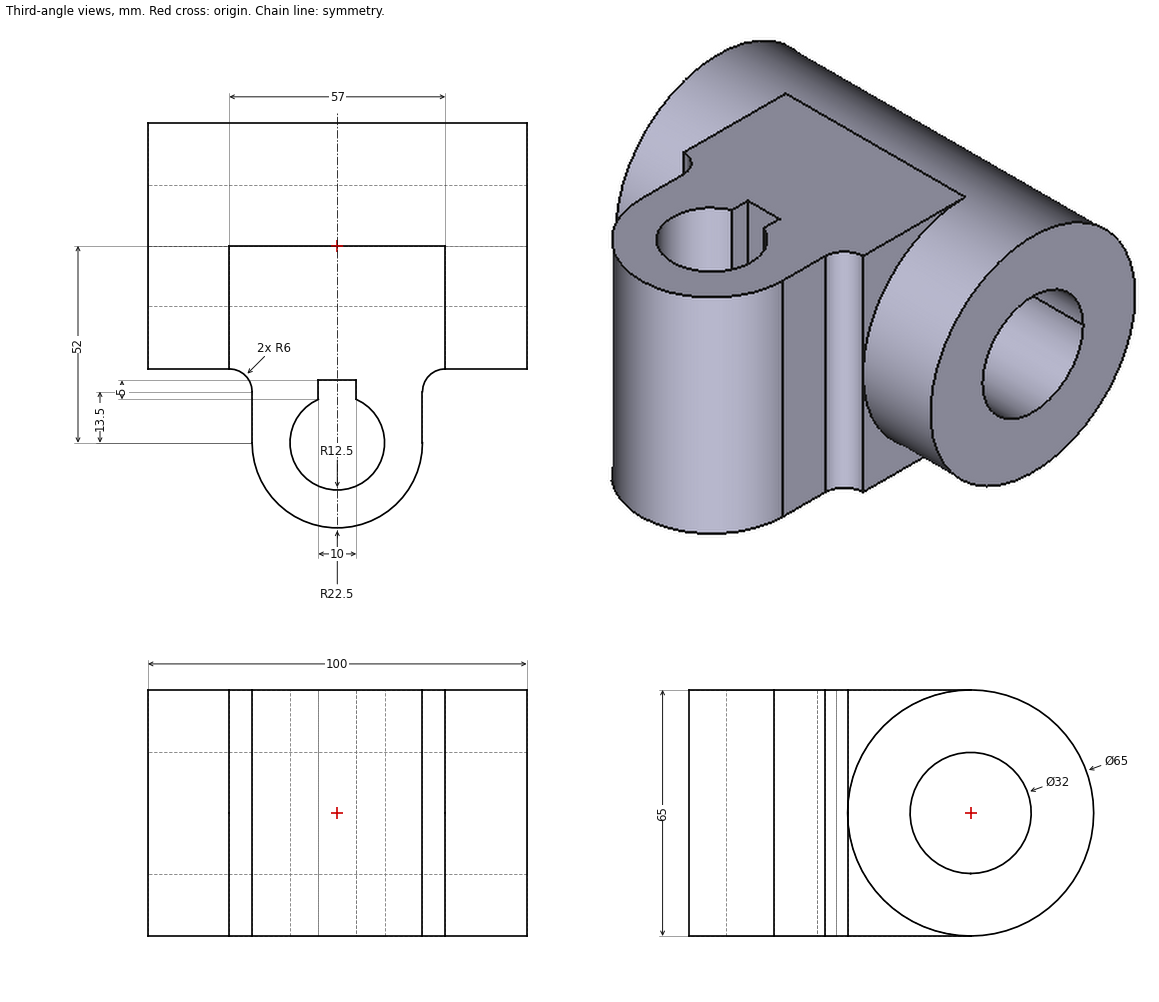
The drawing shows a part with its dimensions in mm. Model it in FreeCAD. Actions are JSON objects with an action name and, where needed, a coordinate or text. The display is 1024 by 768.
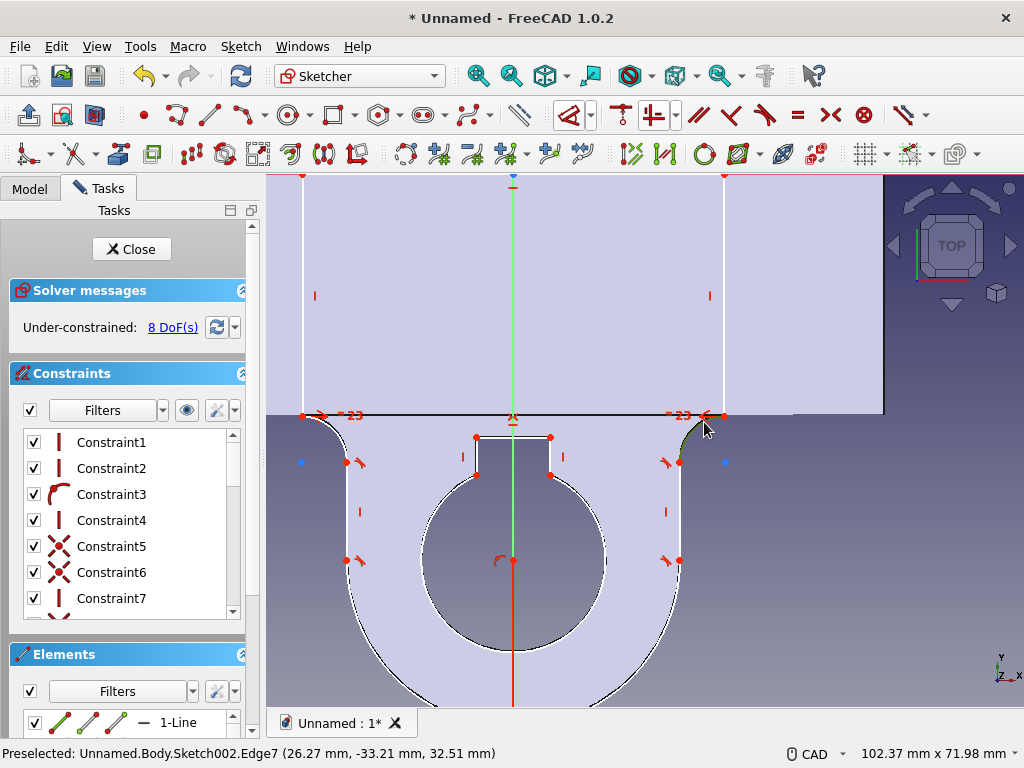
{"action": "key", "text": "k r"}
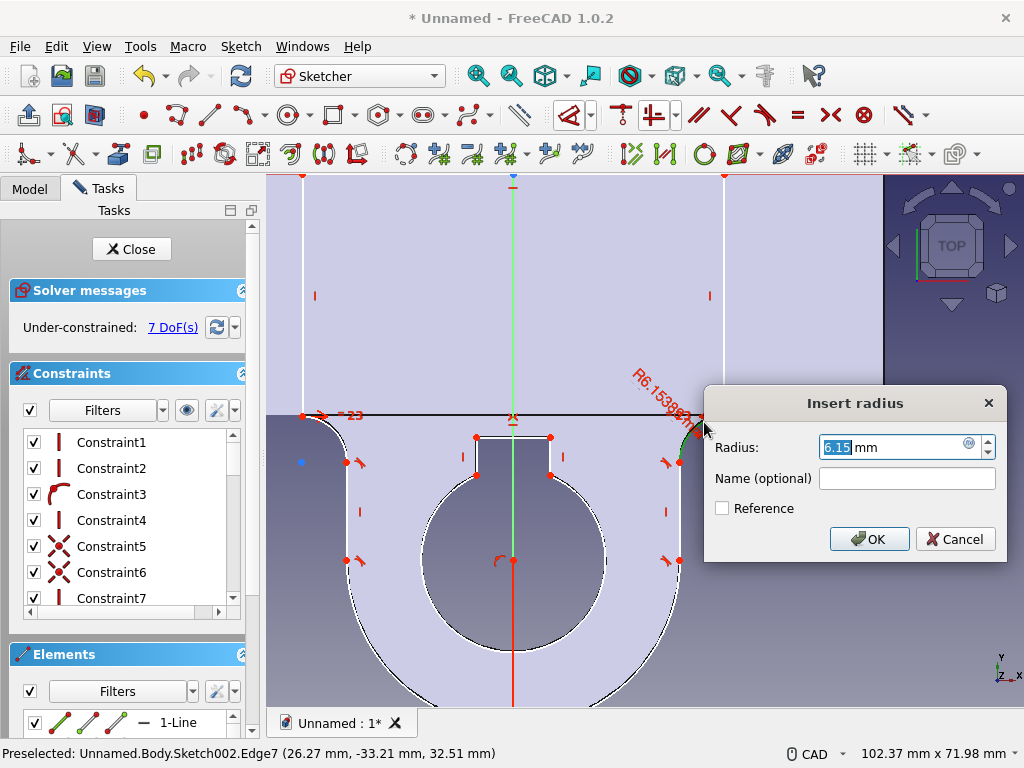
{"action": "type", "text": "6"}
{"action": "key", "text": "Return"}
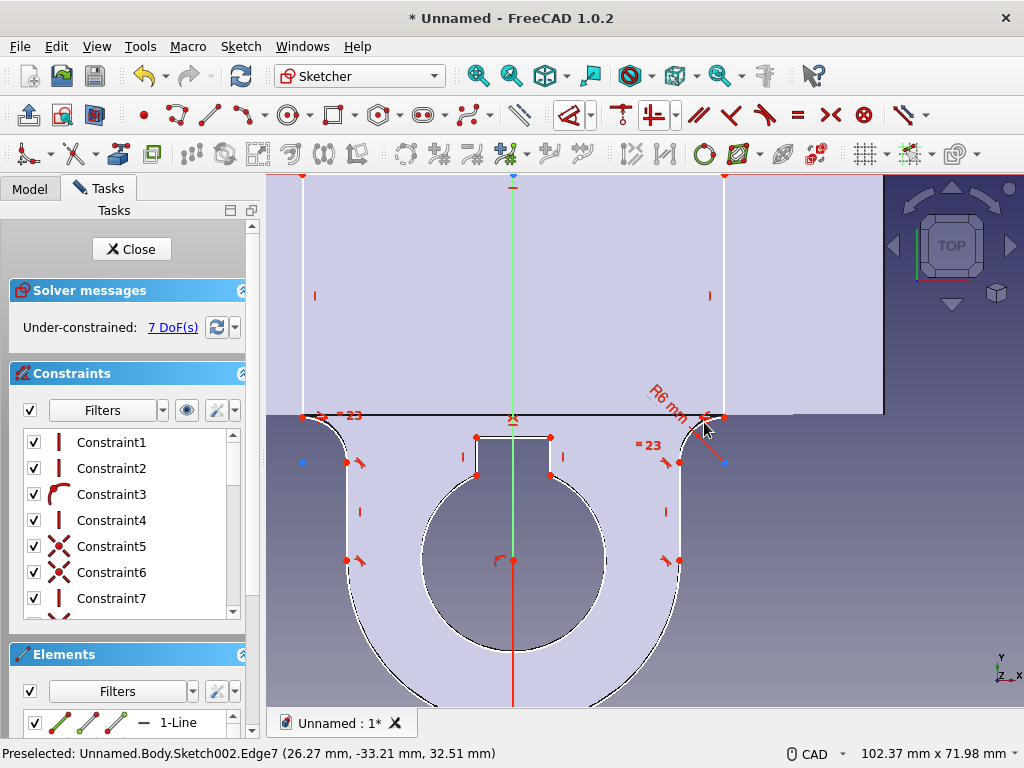
{"action": "left_click", "coordinate": [432, 603]}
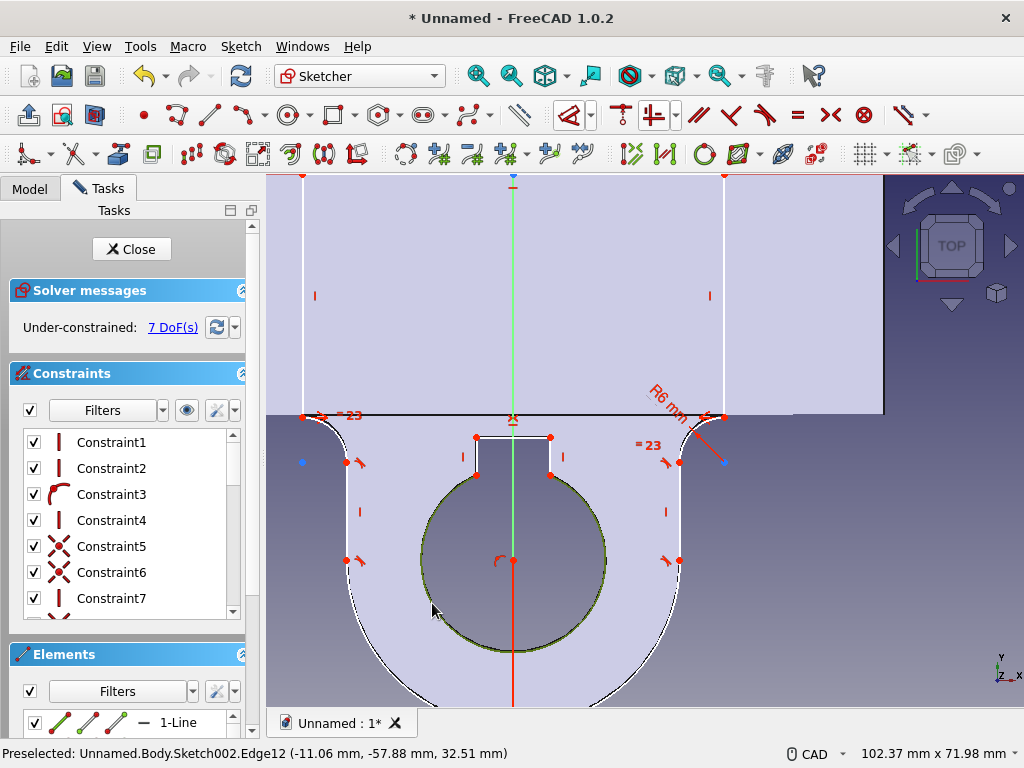
{"action": "left_click", "coordinate": [590, 116]}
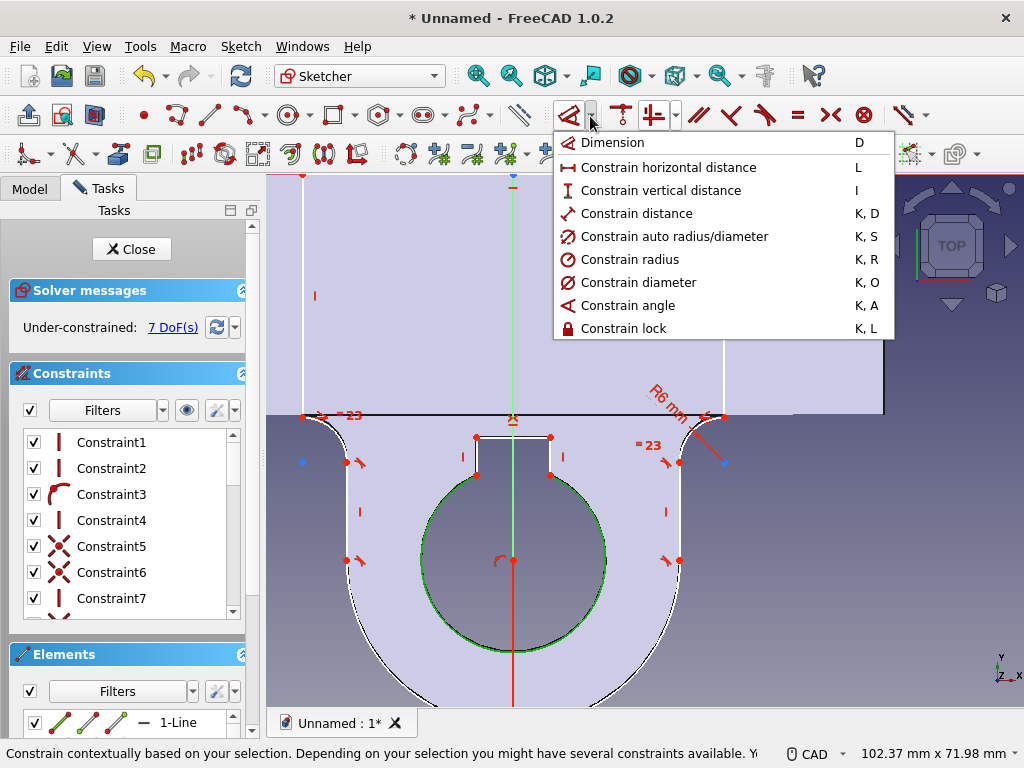
{"action": "left_click", "coordinate": [724, 260]}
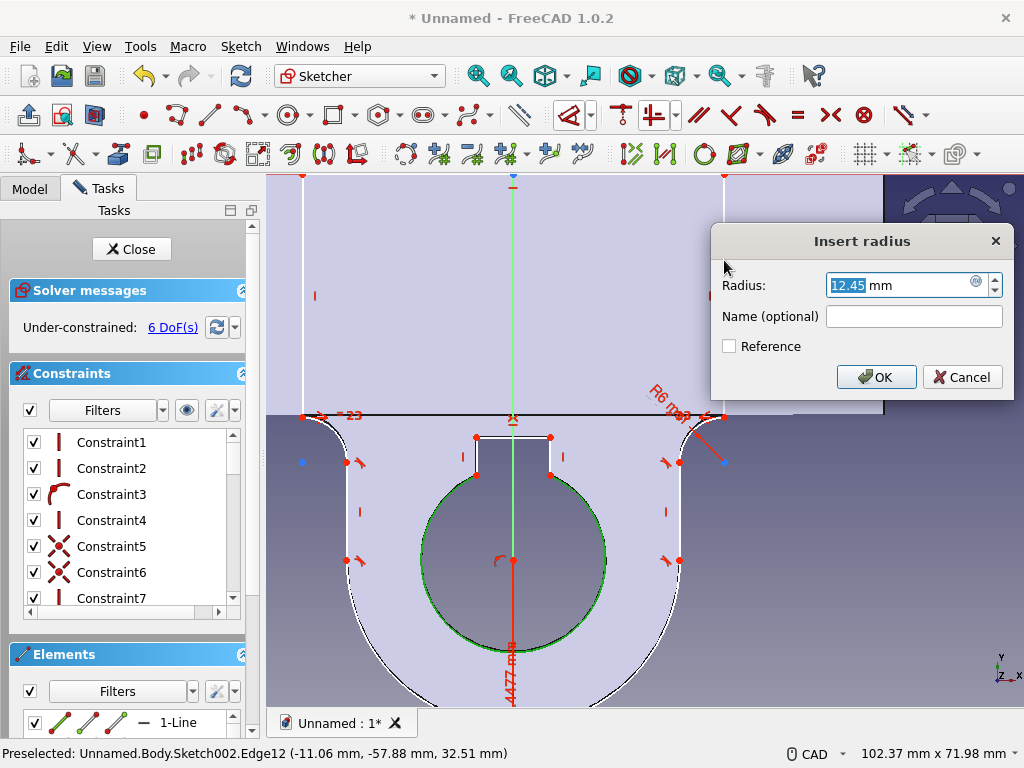
{"action": "type", "text": "12.5"}
{"action": "key", "text": "Return"}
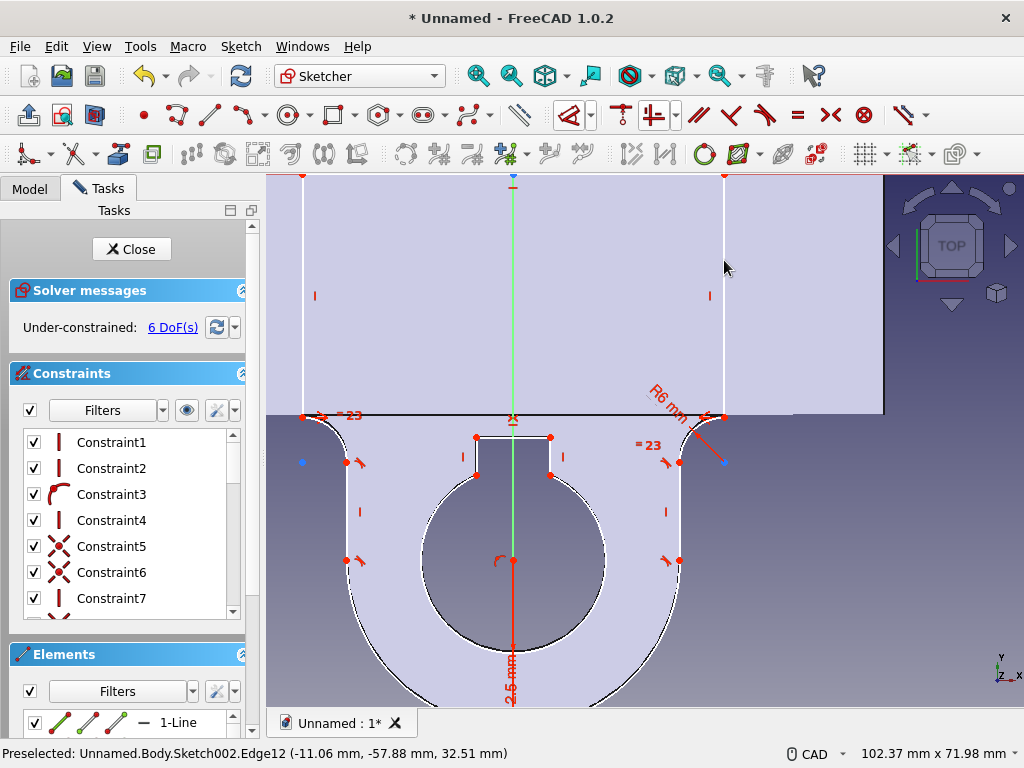
{"action": "left_click", "coordinate": [477, 464]}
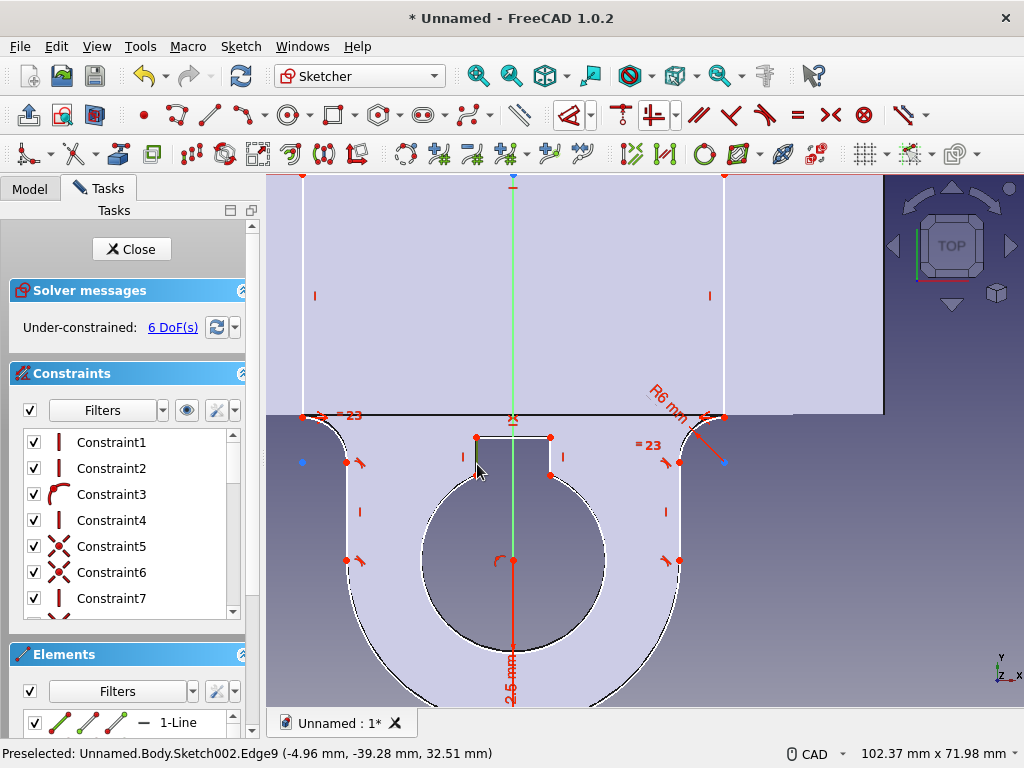
{"action": "key", "text": "i"}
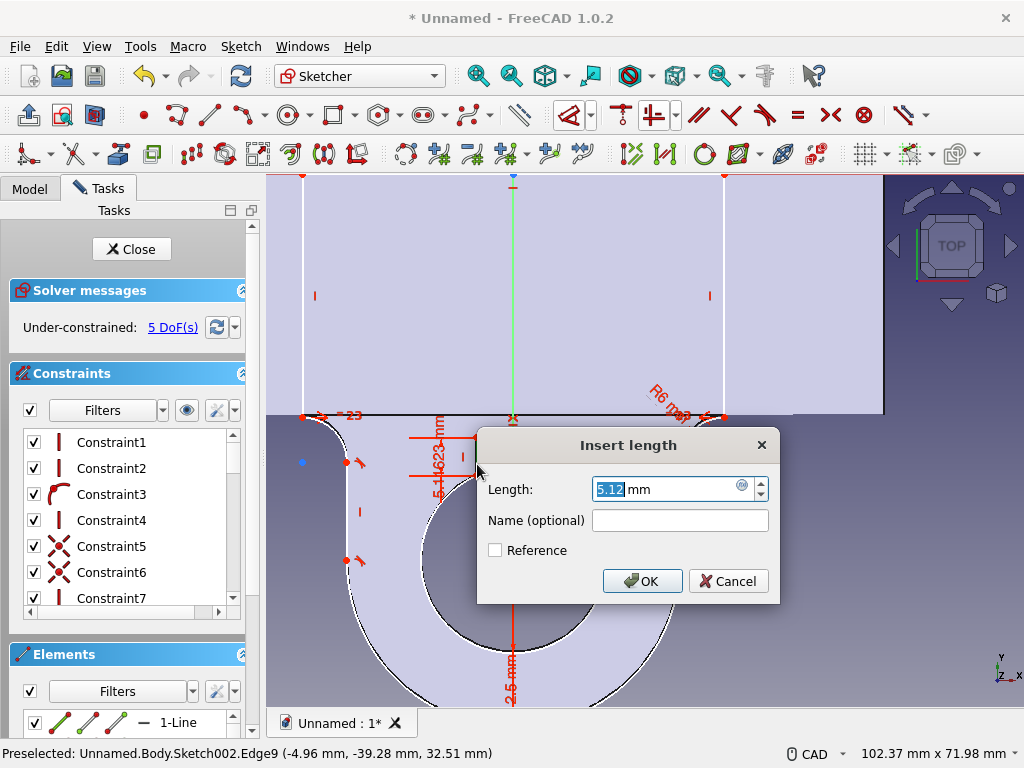
{"action": "type", "text": "5"}
{"action": "key", "text": "Return"}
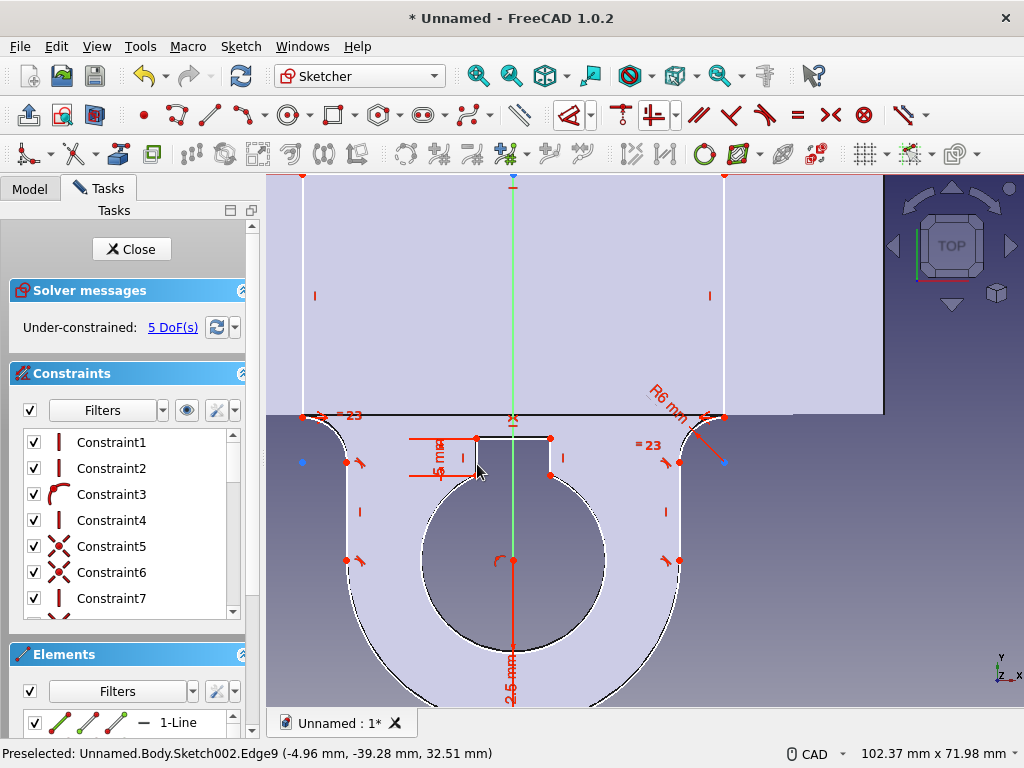
{"action": "scroll", "coordinate": [550, 450], "scroll_direction": "up", "scroll_amount": 2}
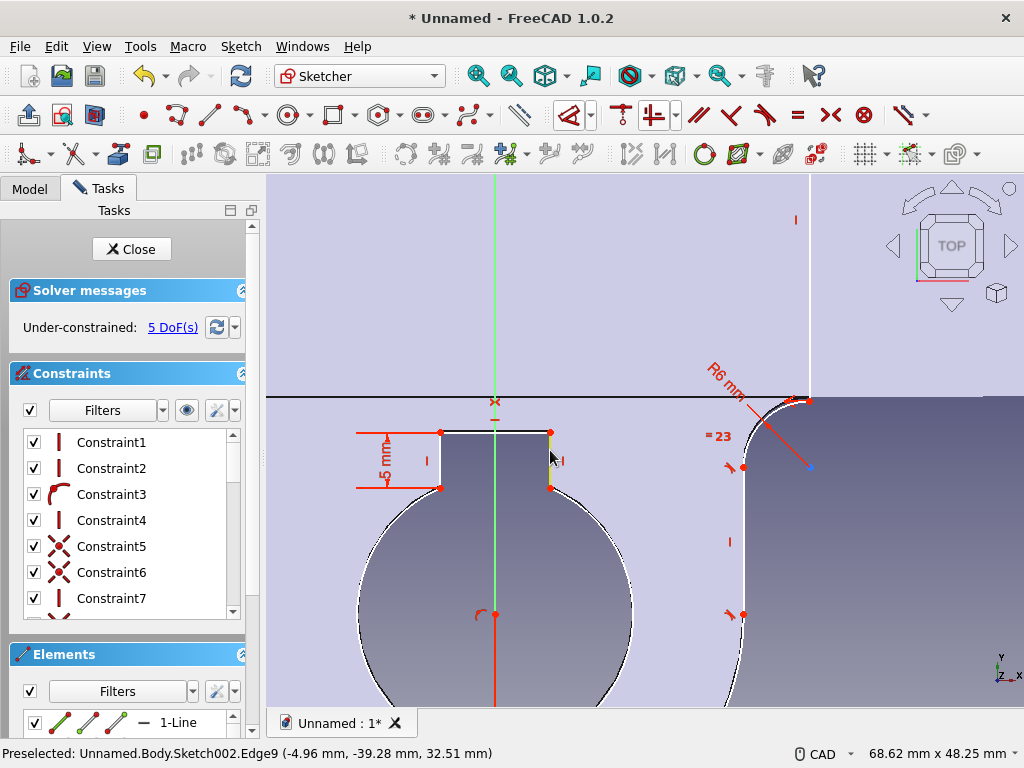
{"action": "left_click", "coordinate": [550, 450]}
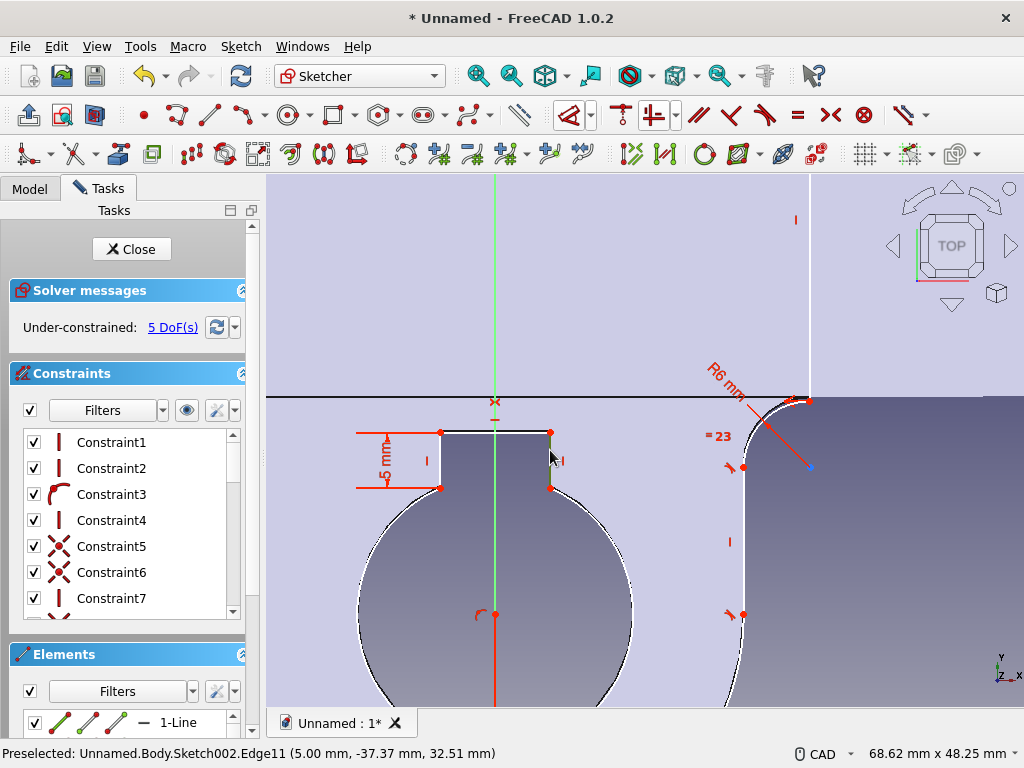
{"action": "key", "text": "i"}